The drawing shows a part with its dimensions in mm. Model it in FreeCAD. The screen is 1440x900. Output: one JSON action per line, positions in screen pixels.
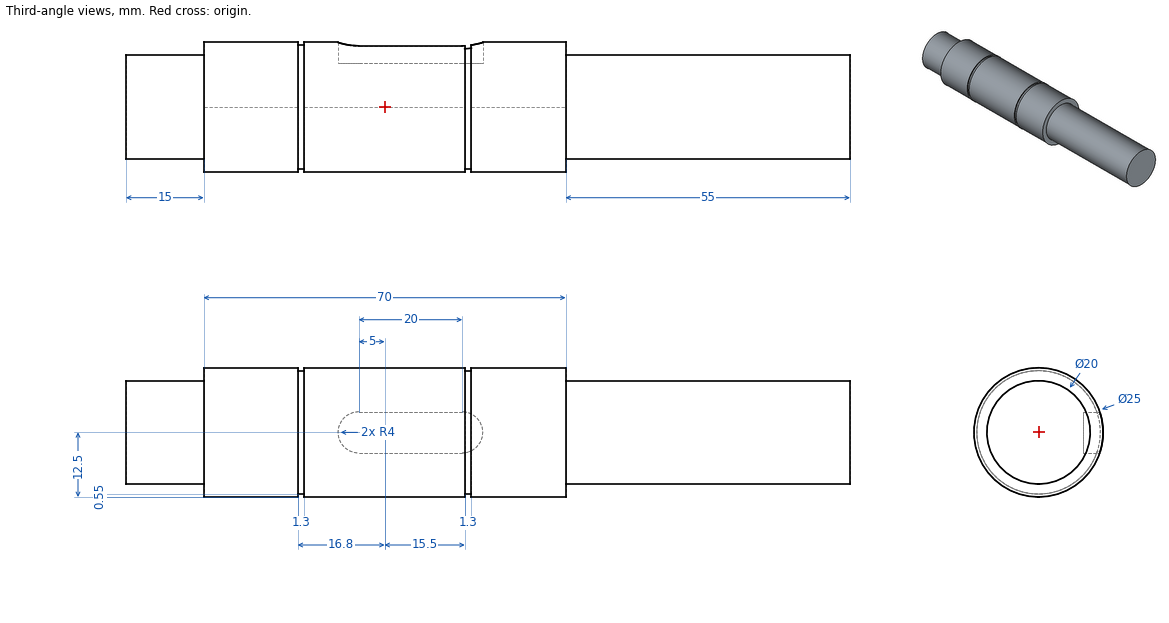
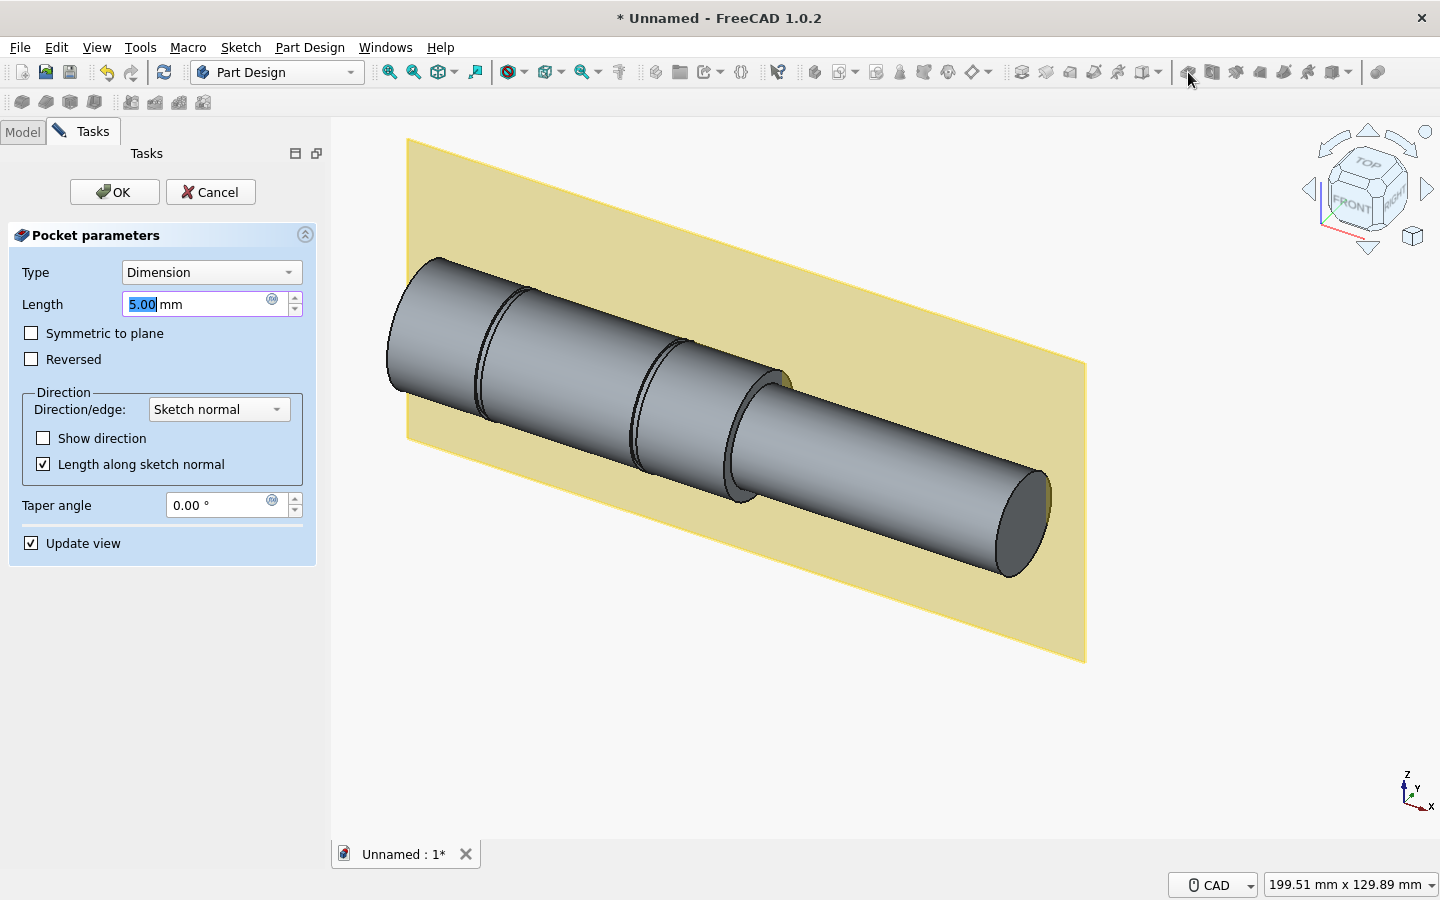
{"action": "left_click", "coordinate": [212, 272]}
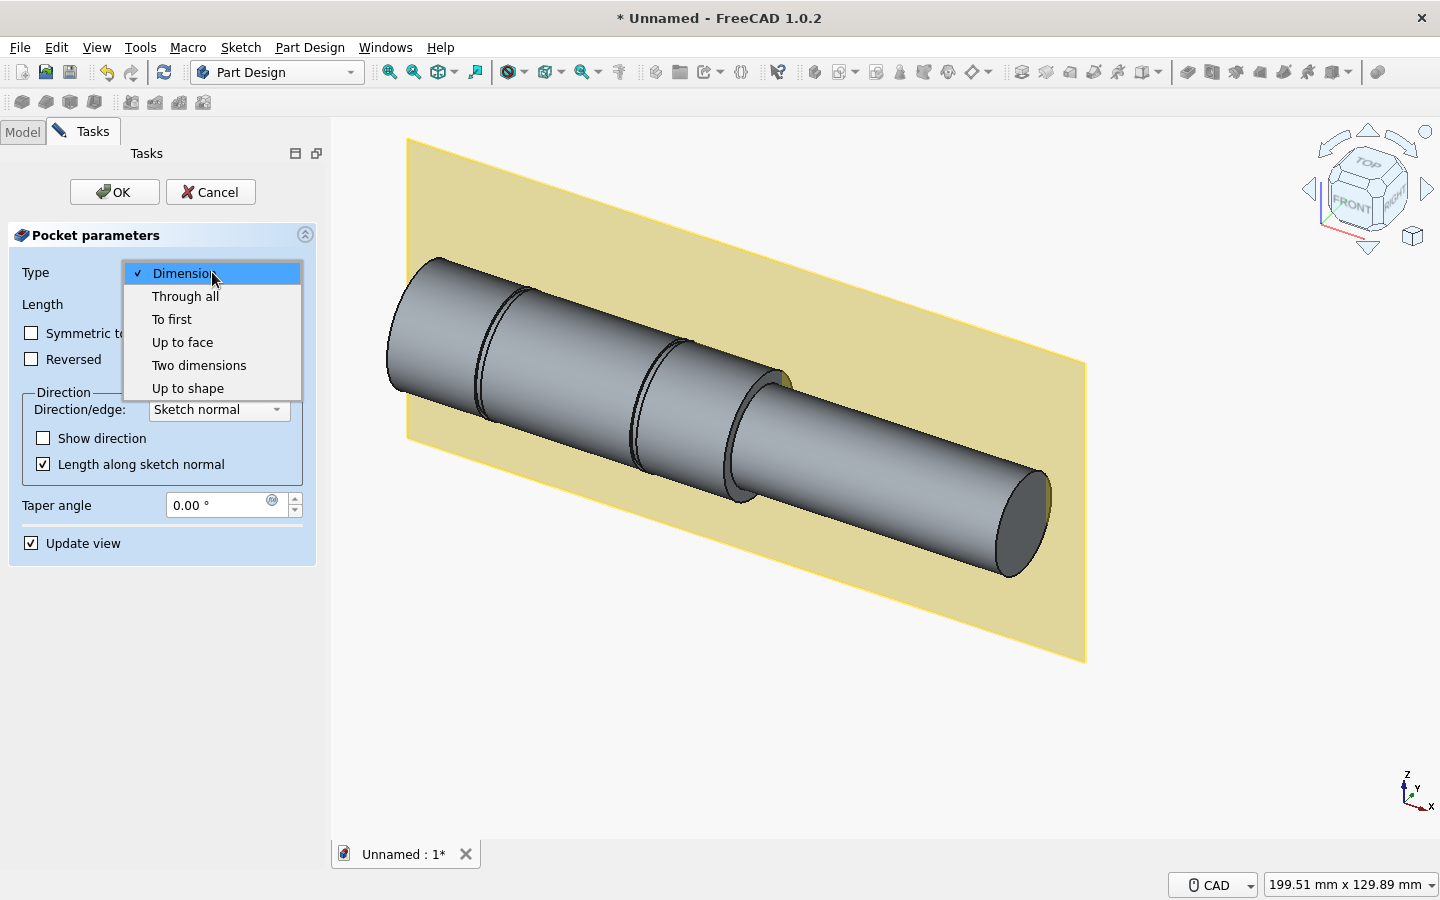
{"action": "left_click", "coordinate": [212, 296]}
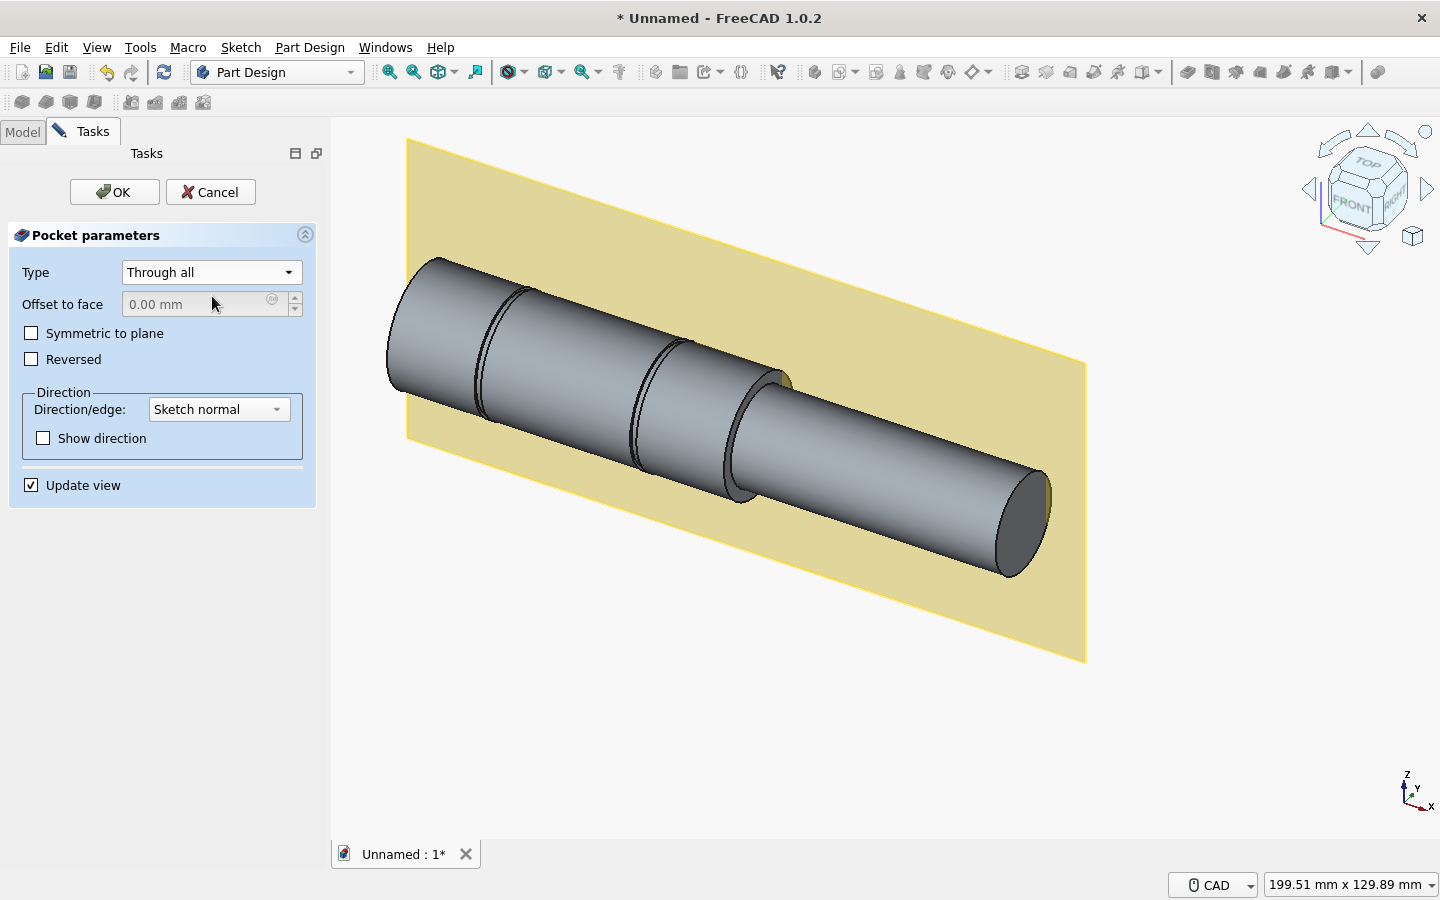
{"action": "left_click", "coordinate": [115, 192]}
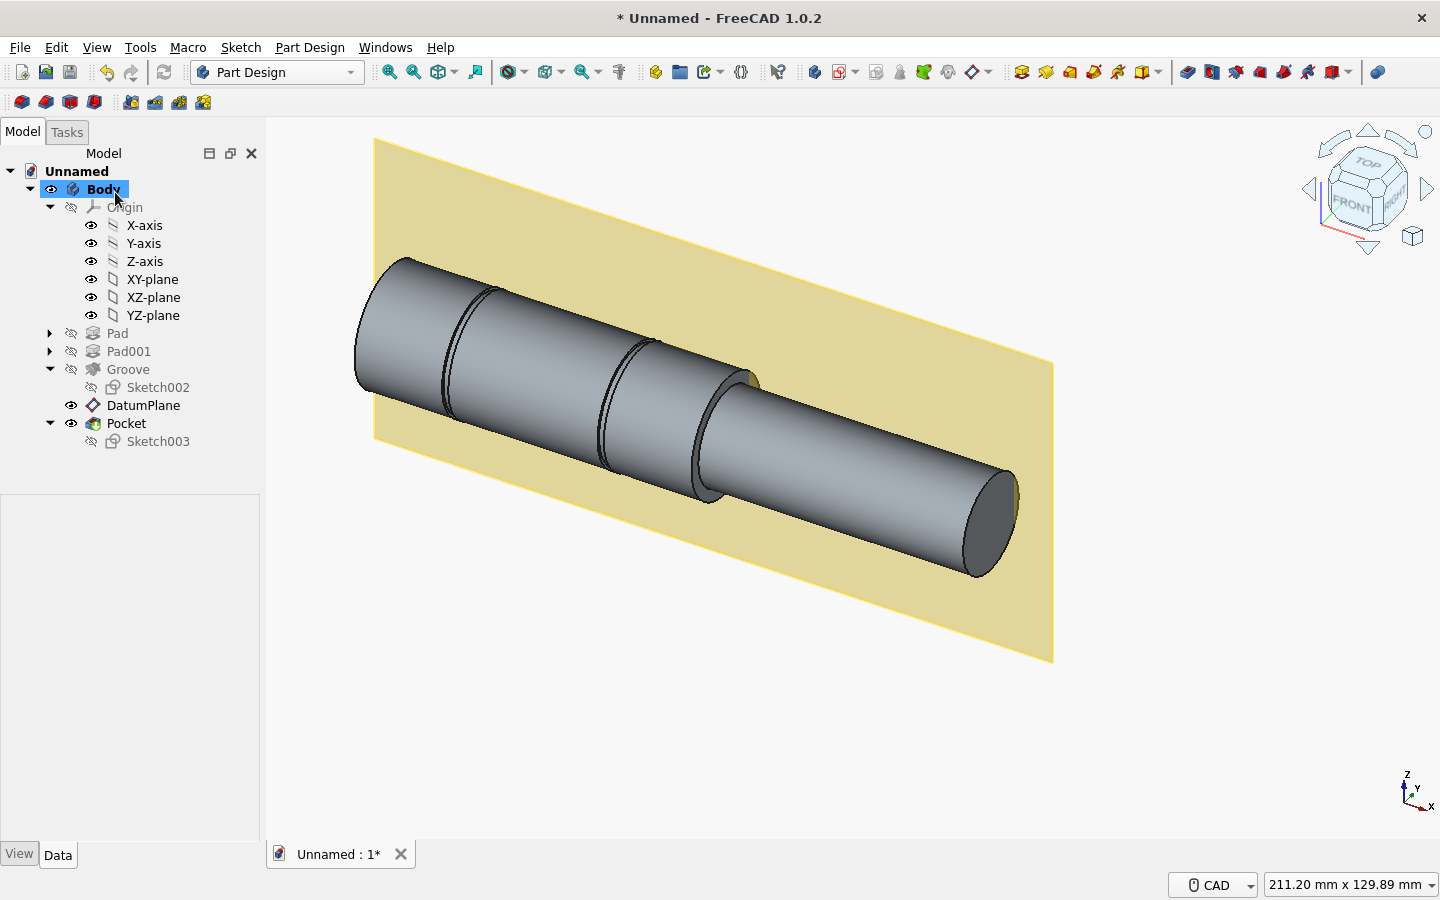
{"action": "left_click", "coordinate": [116, 405]}
{"action": "key", "text": "space"}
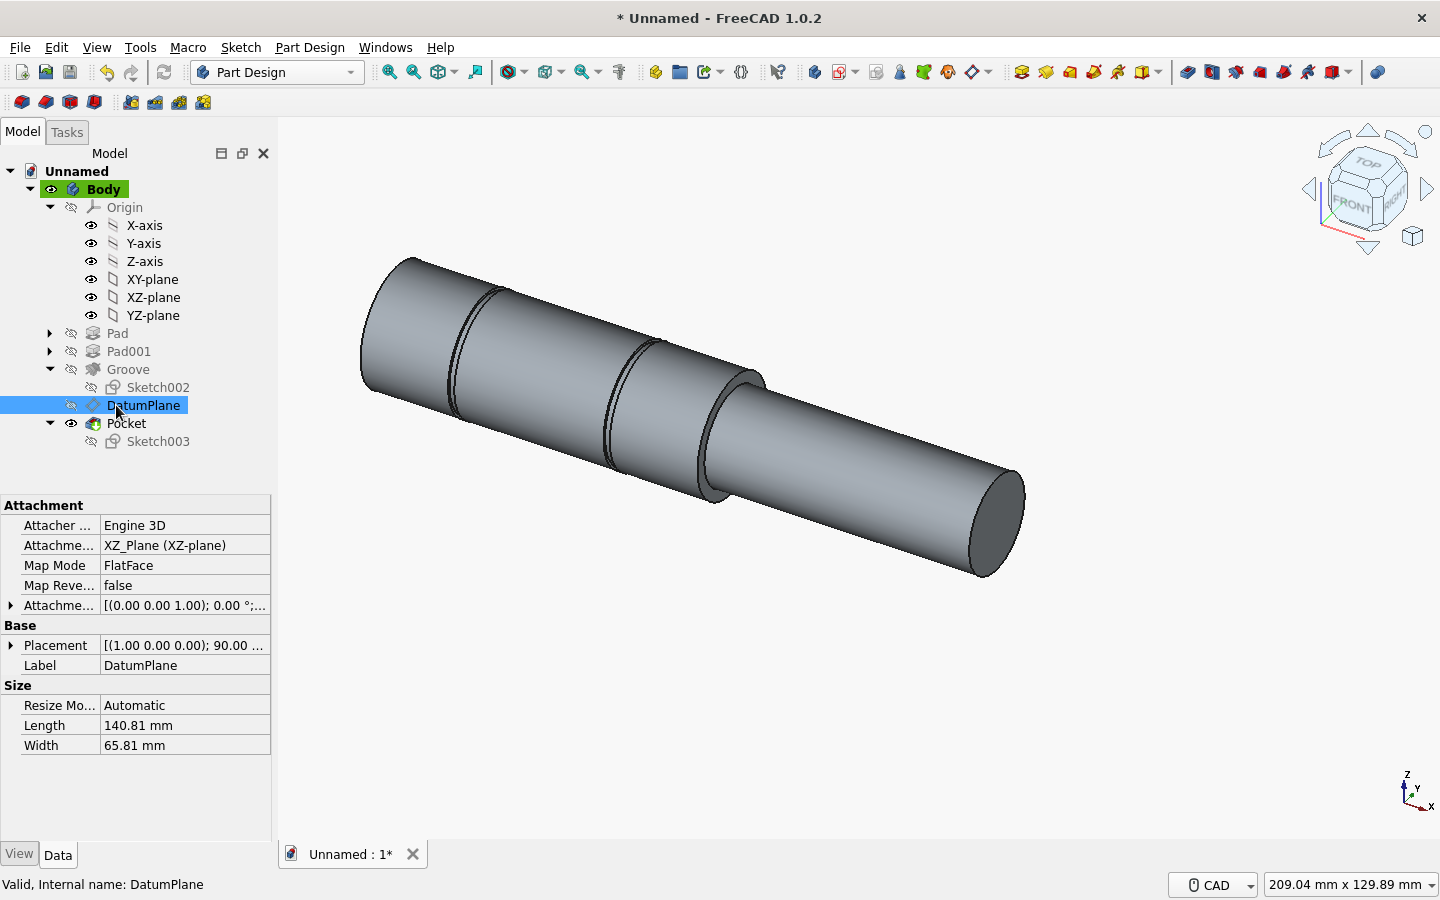
{"action": "left_click", "coordinate": [136, 315]}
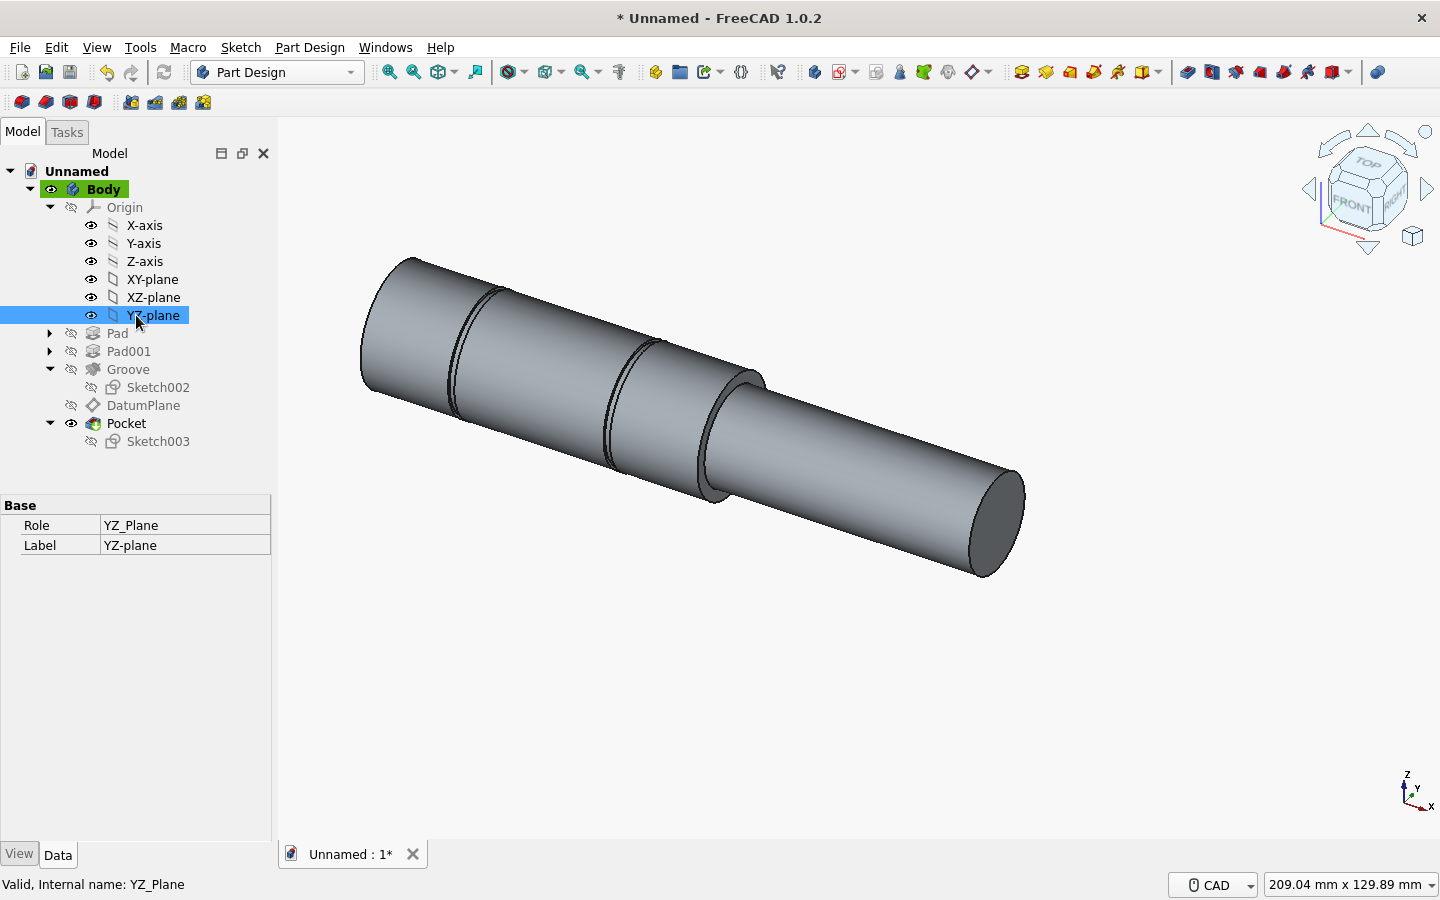
{"action": "left_click", "coordinate": [972, 72]}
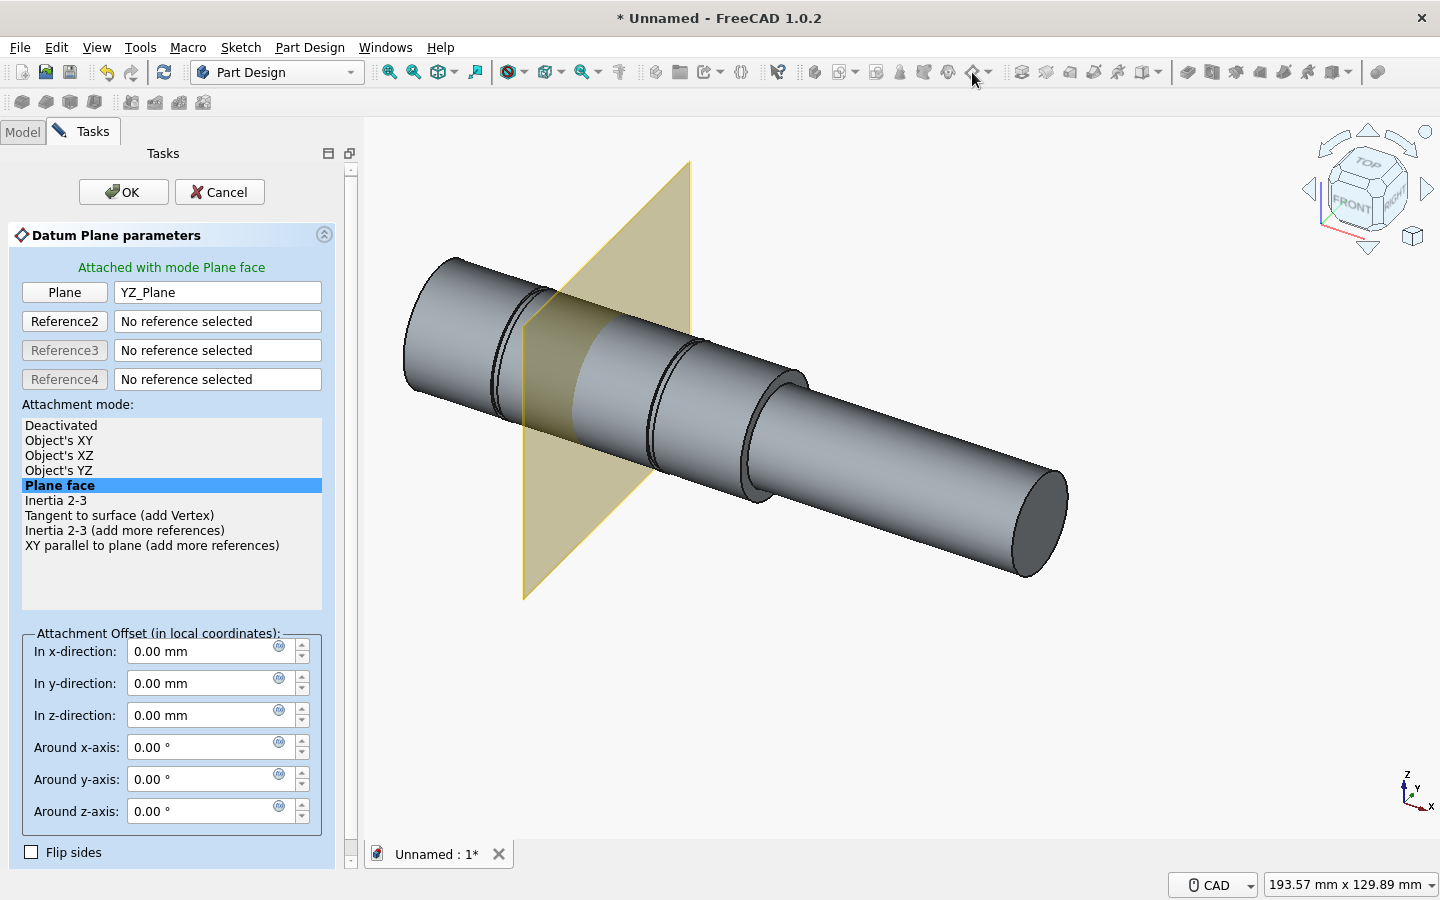
{"action": "triple_click", "coordinate": [210, 715]}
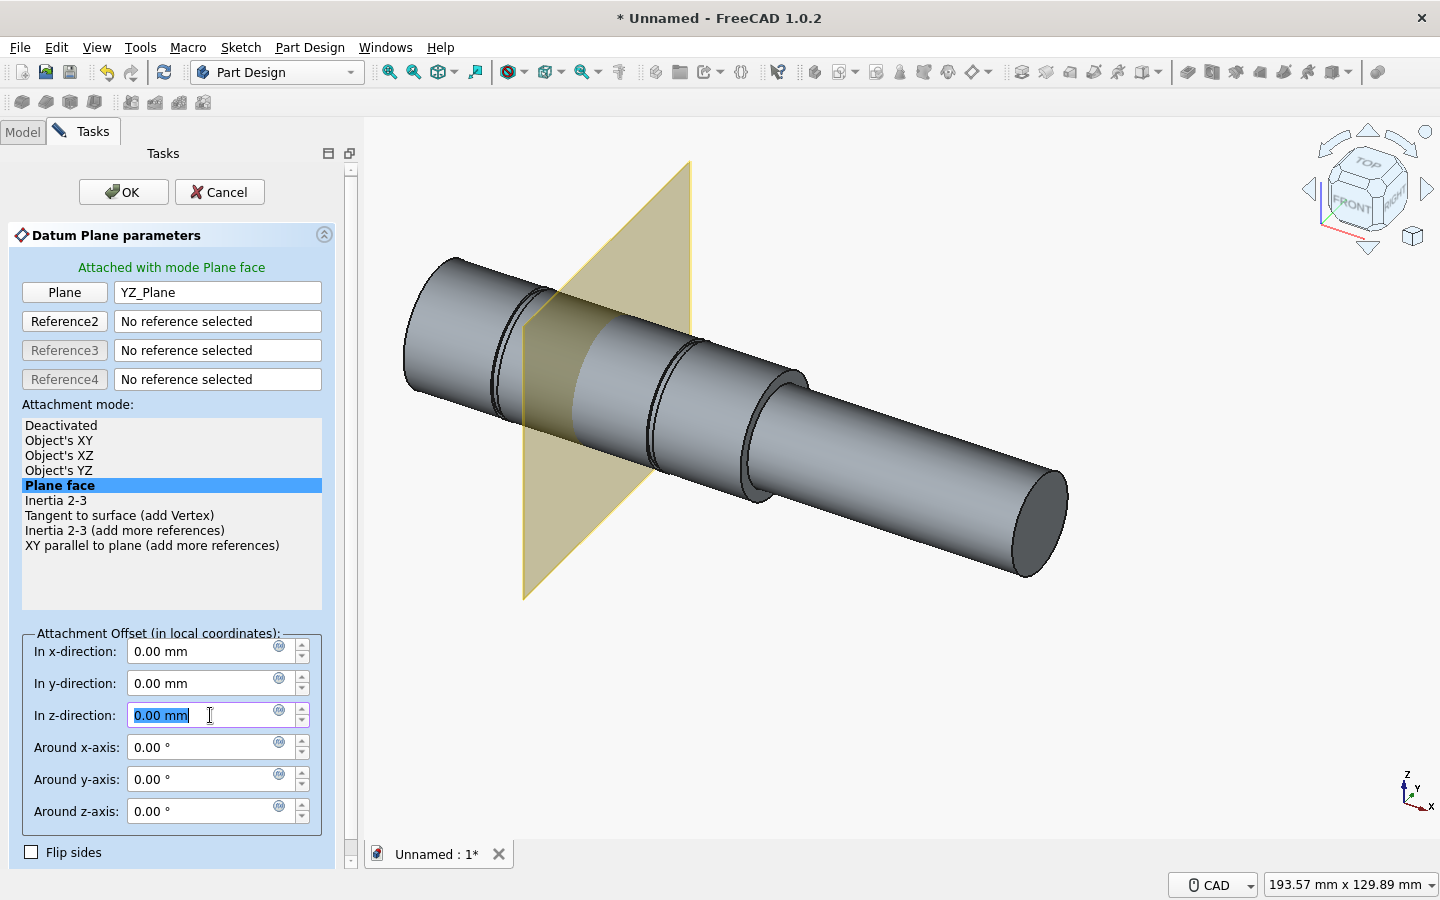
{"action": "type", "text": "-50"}
{"action": "key", "text": "Tab"}